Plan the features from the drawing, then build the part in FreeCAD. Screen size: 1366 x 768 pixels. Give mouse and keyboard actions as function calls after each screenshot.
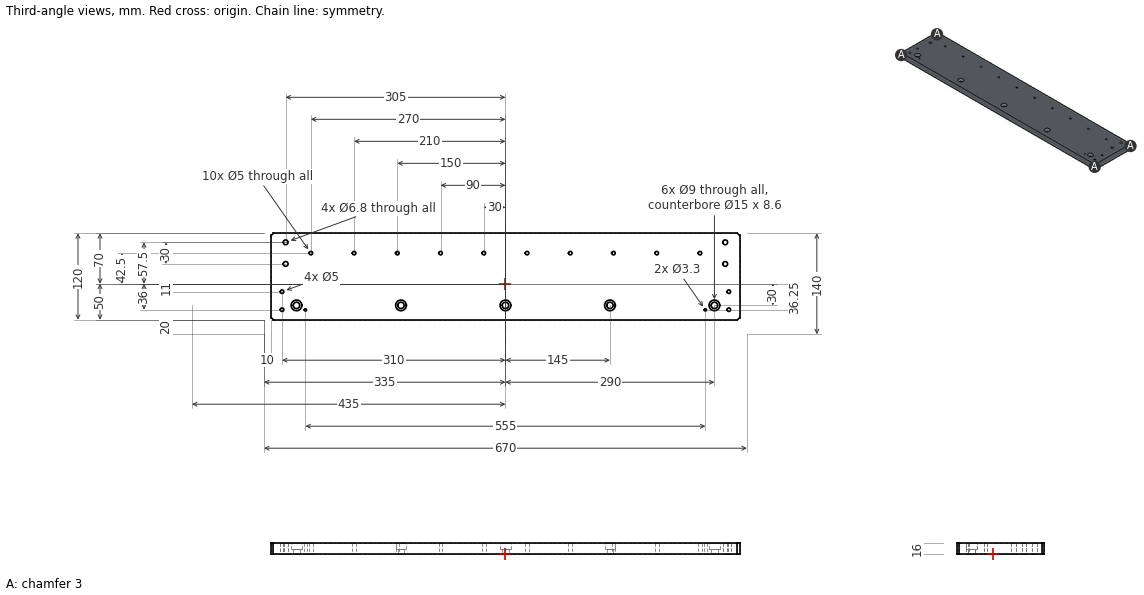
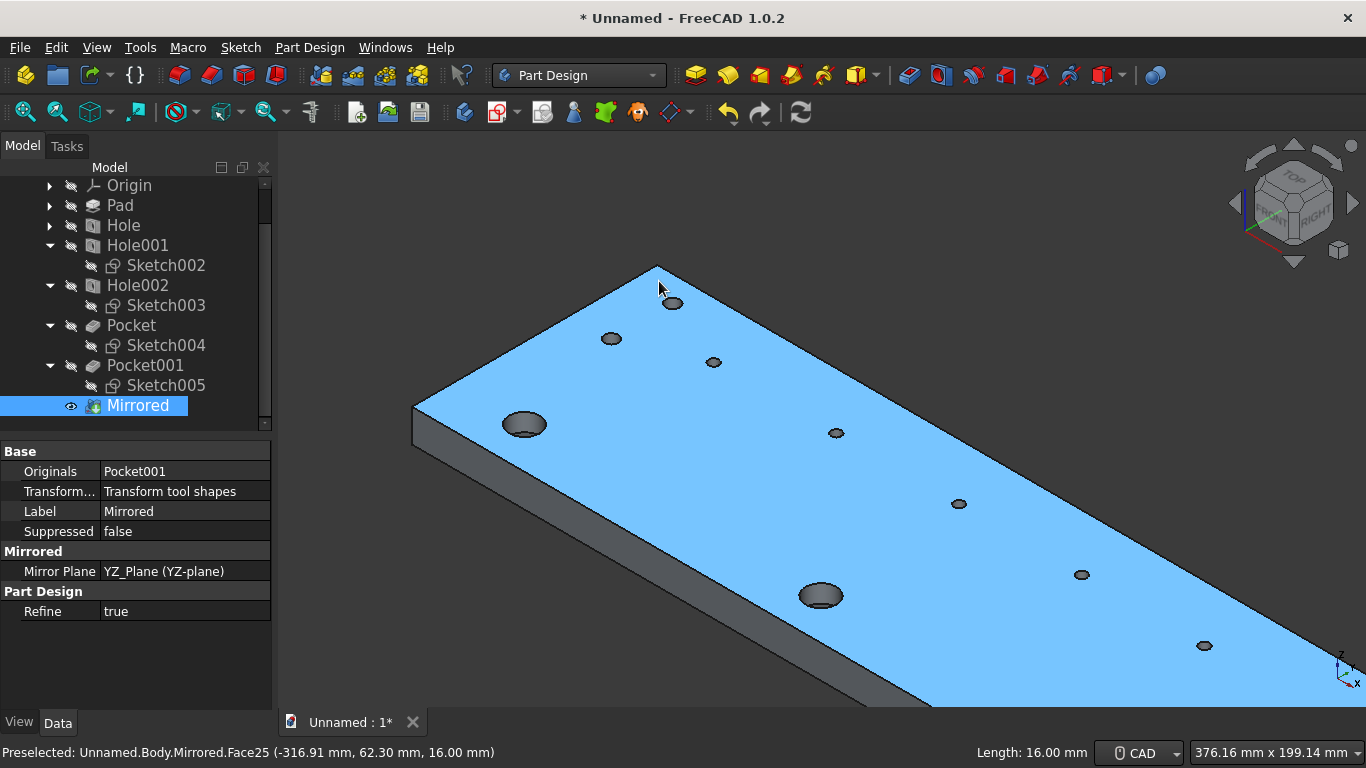
click(26, 112)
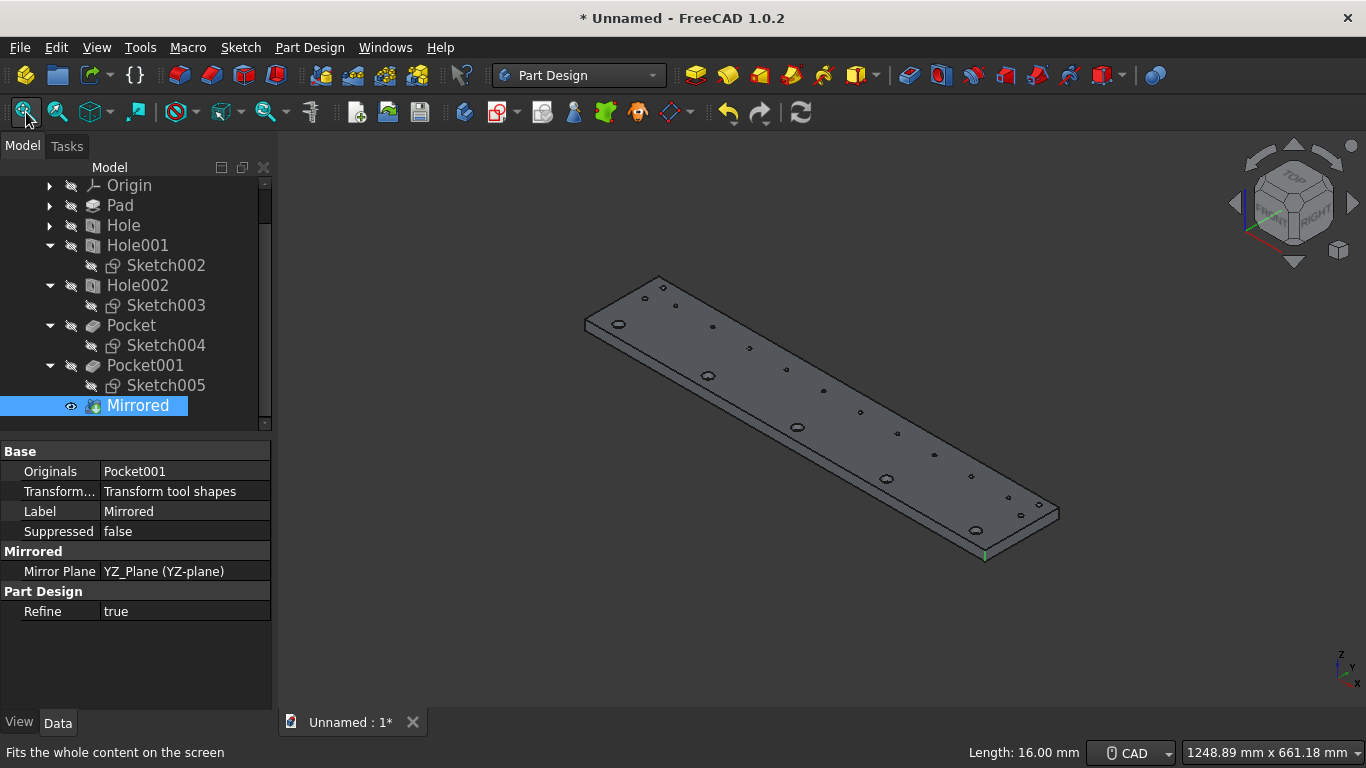
key(2)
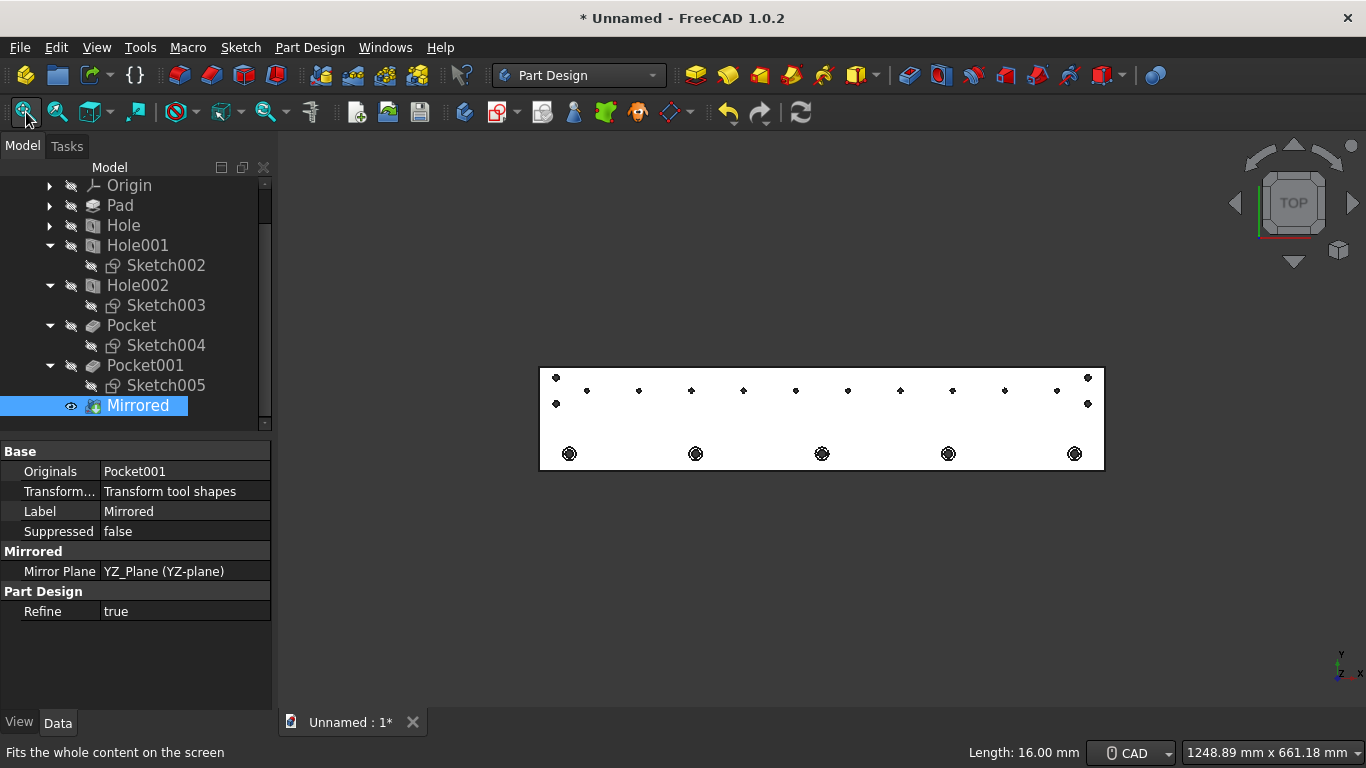
scroll(539, 366, up, 6)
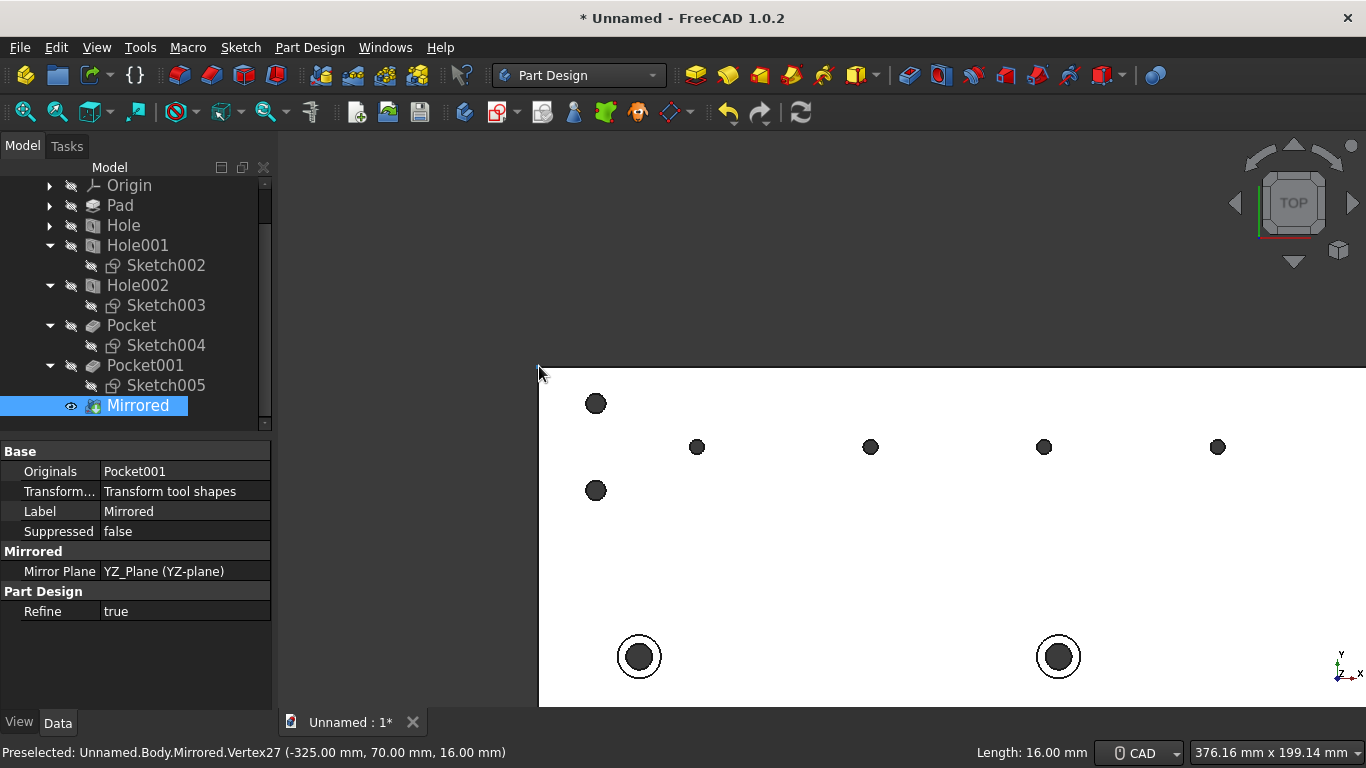
click(26, 112)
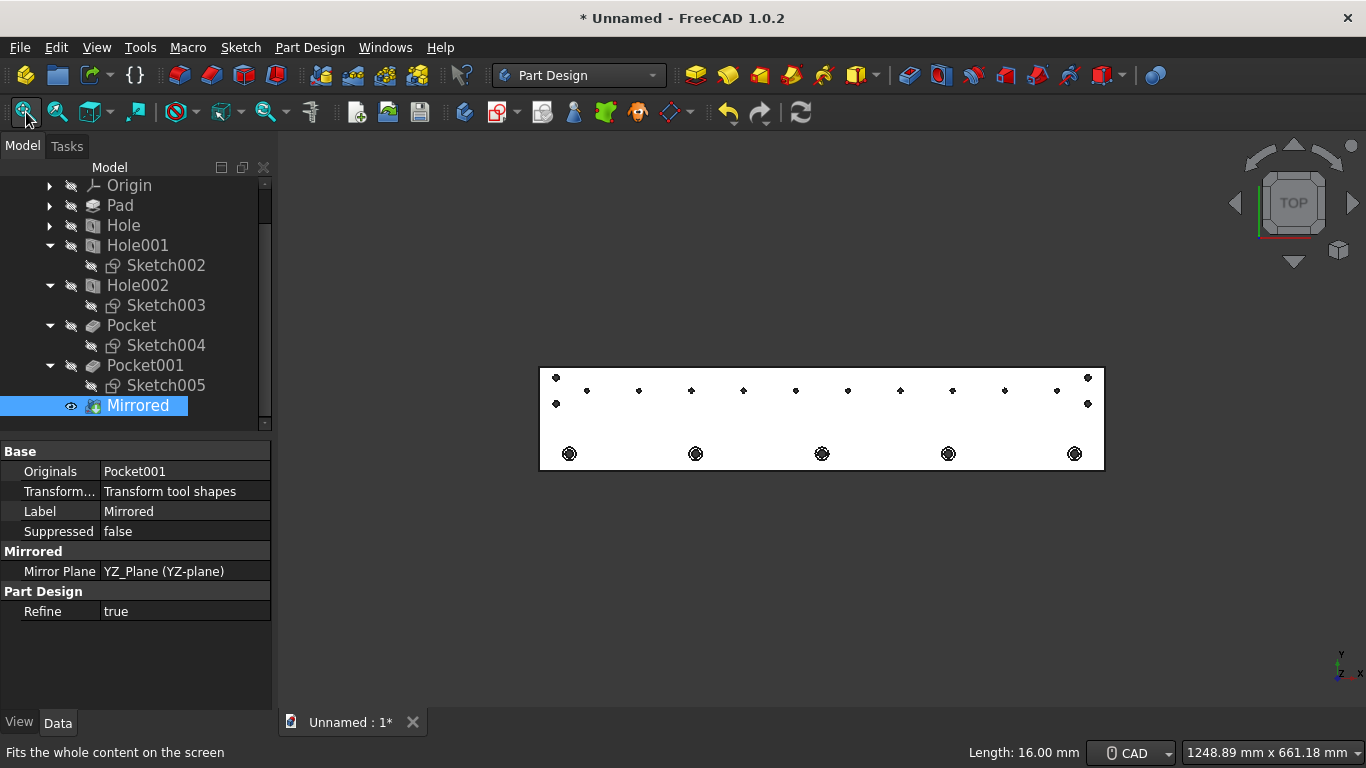
key(1)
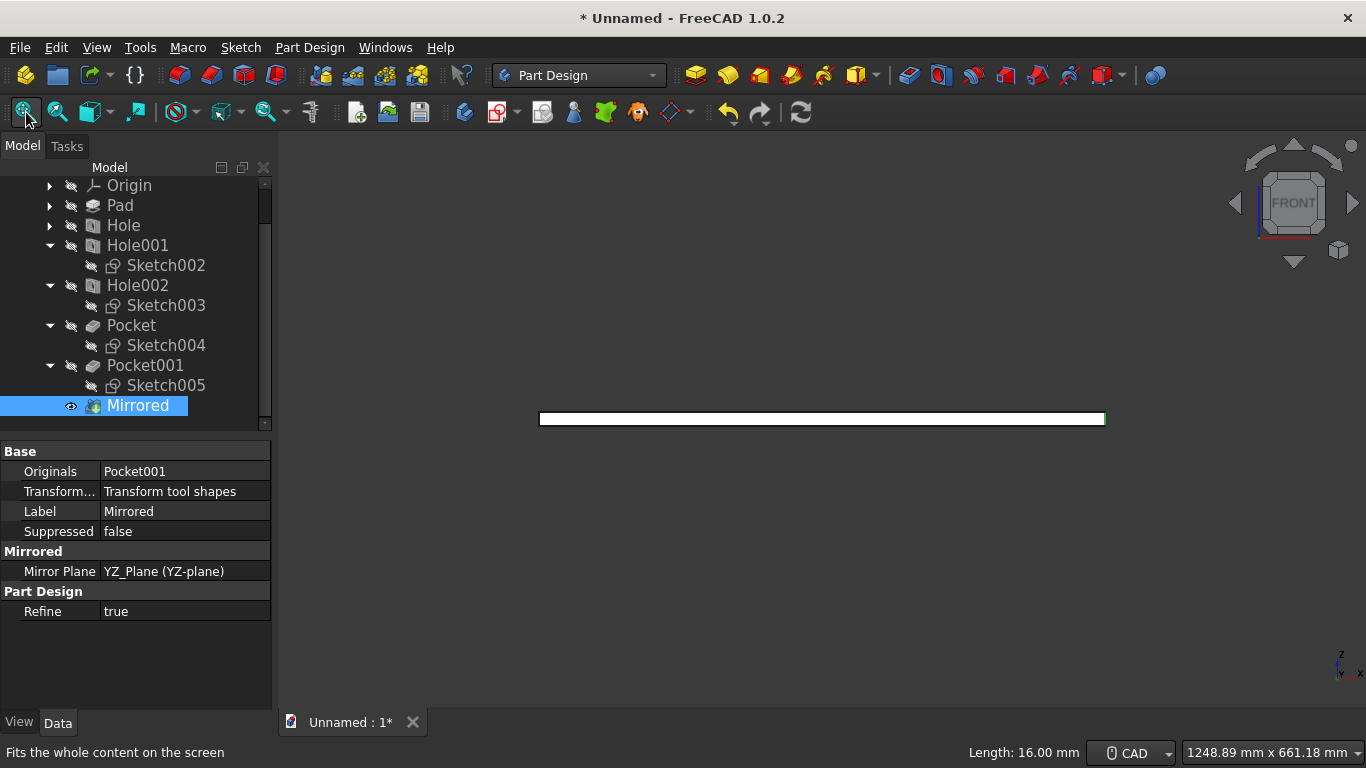
click(539, 418, ctrl)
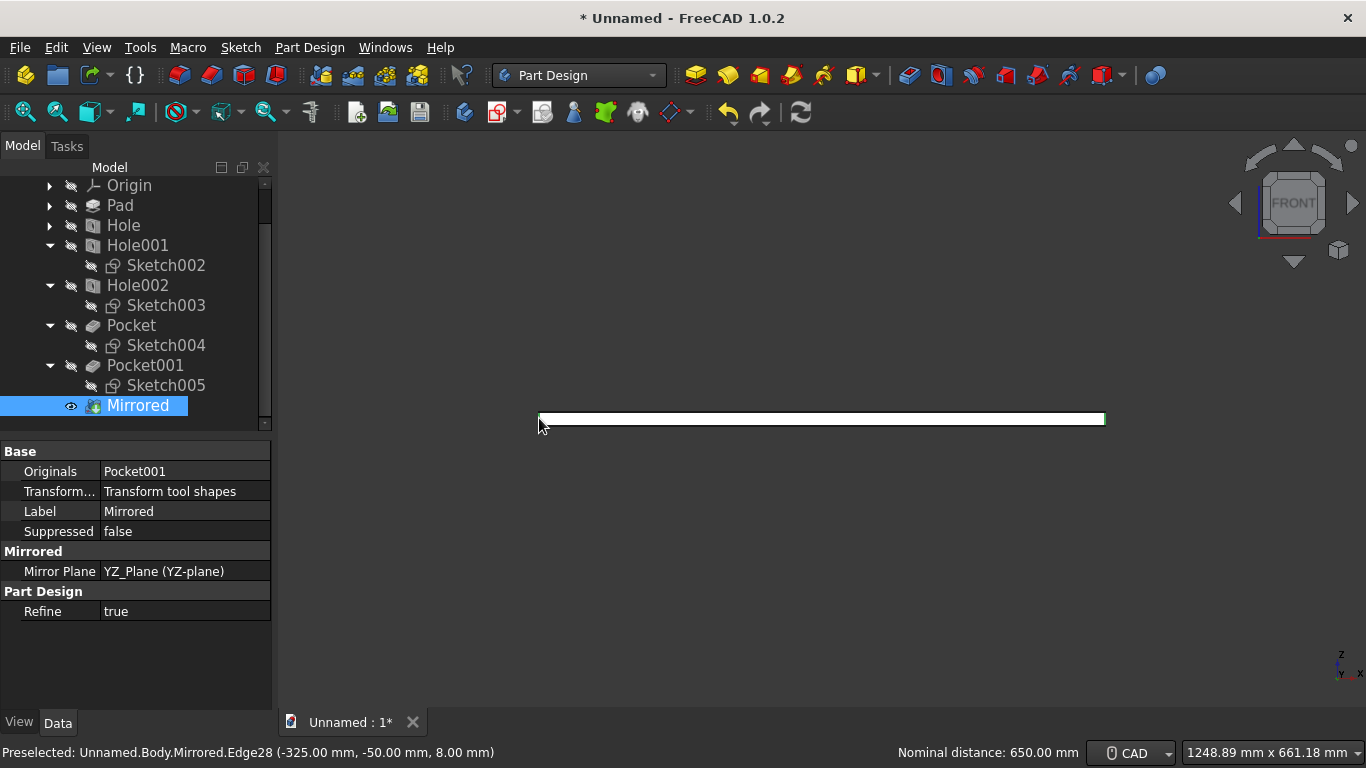
scroll(539, 418, up, 6)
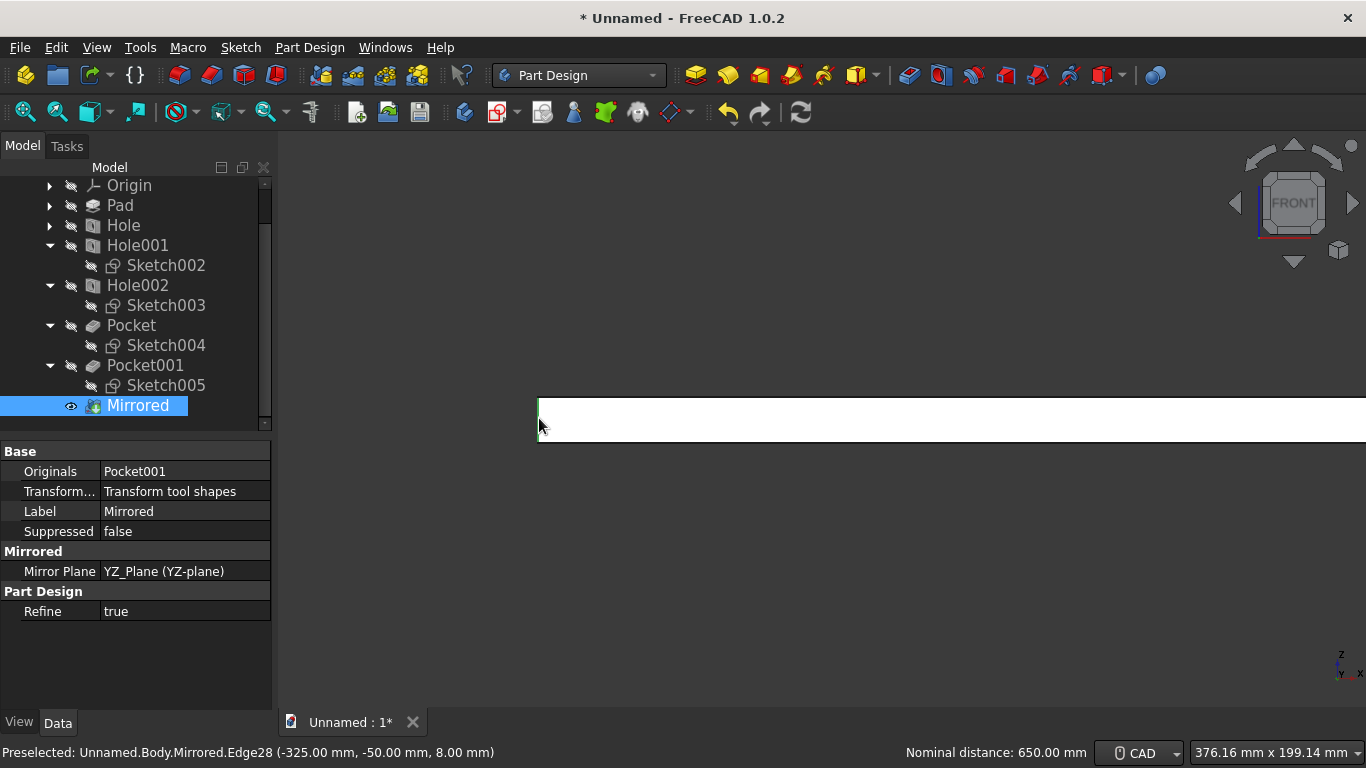
click(26, 112)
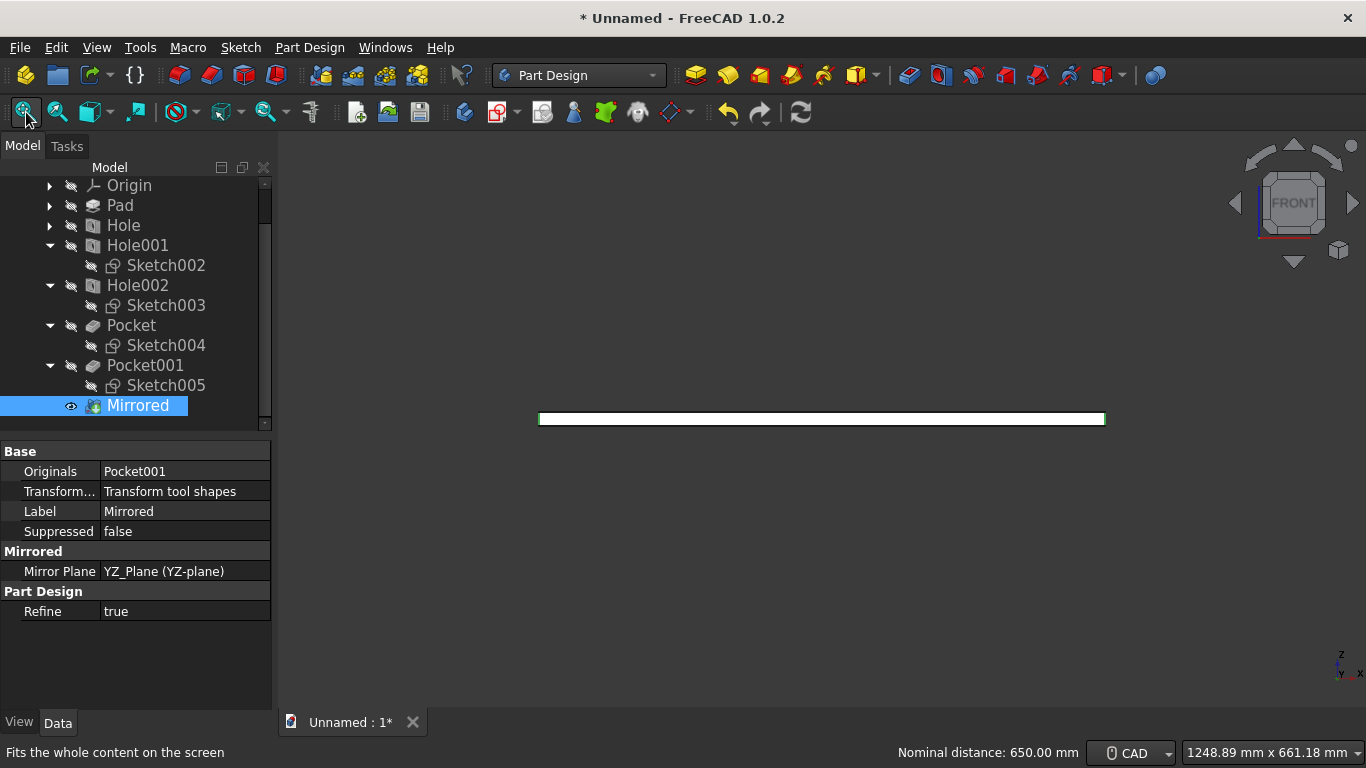
key(3)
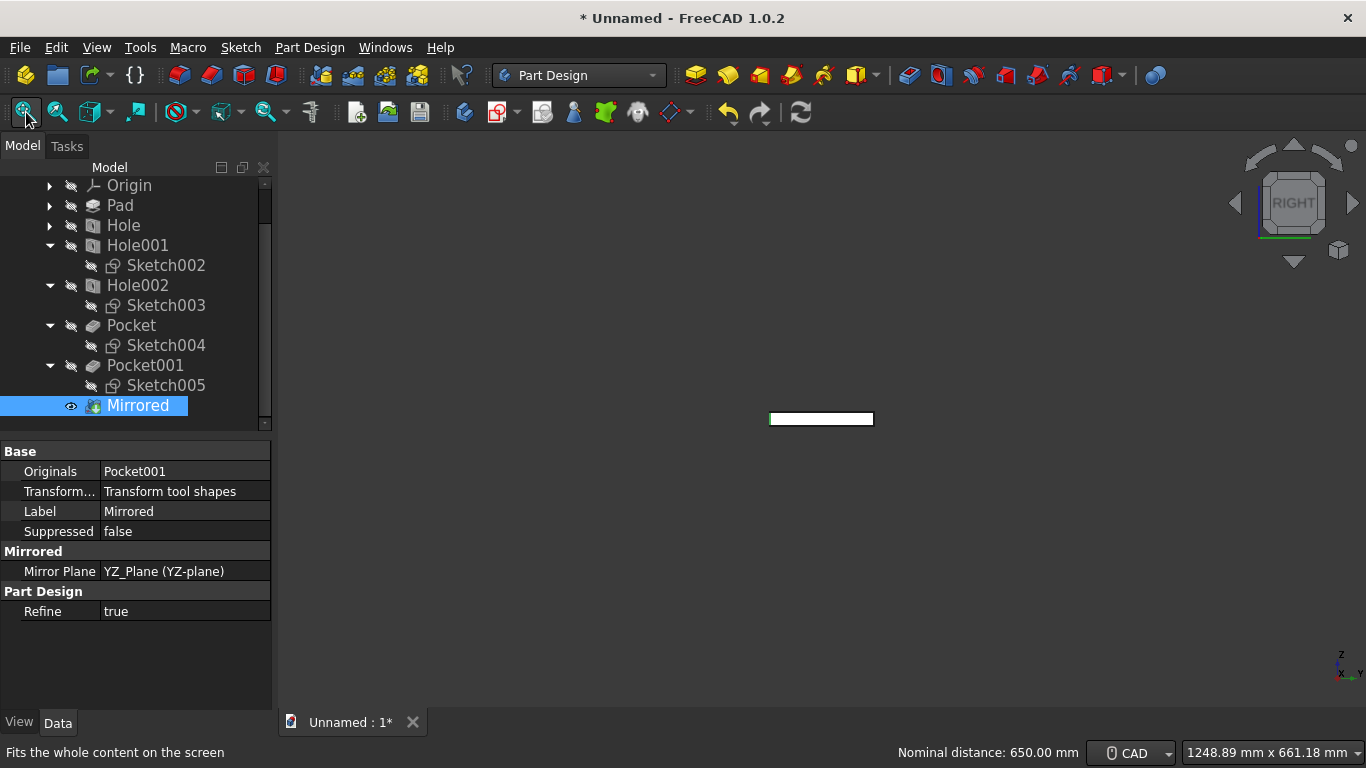
click(26, 112)